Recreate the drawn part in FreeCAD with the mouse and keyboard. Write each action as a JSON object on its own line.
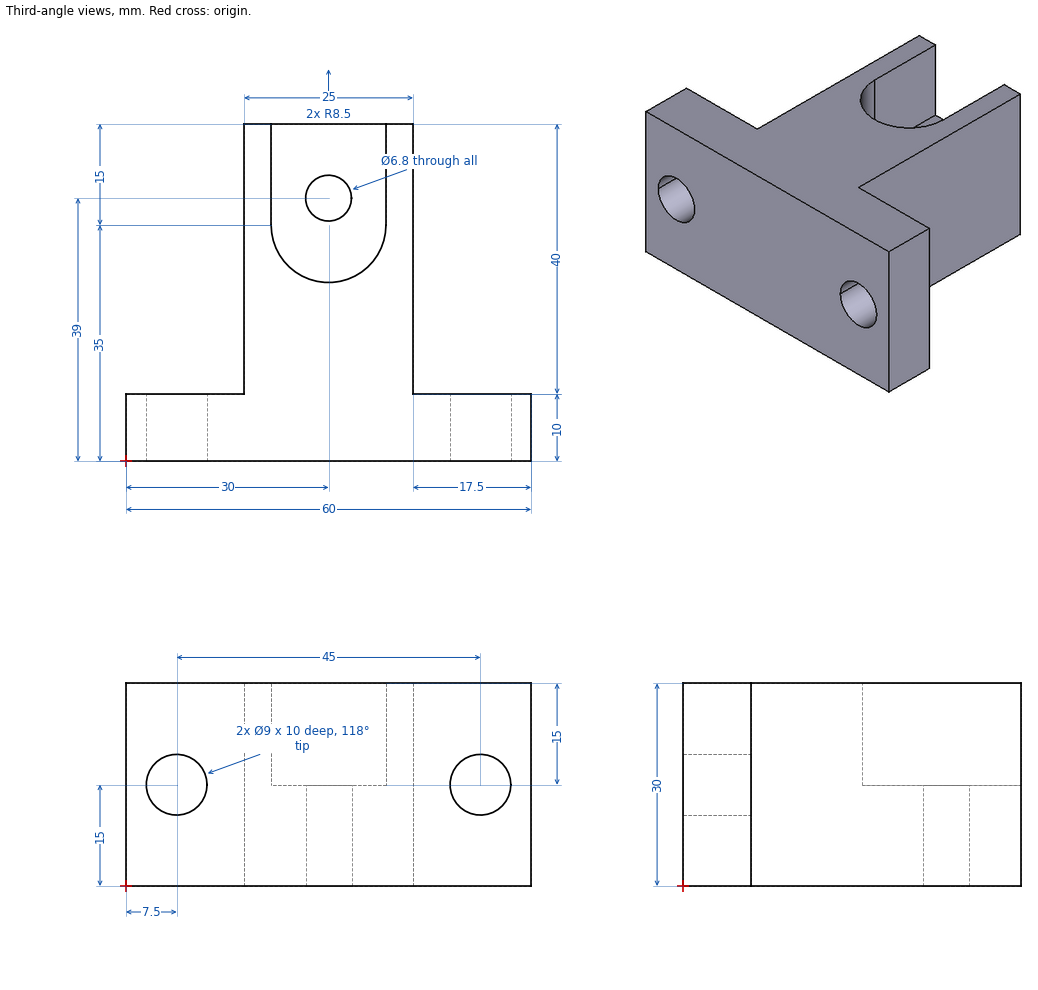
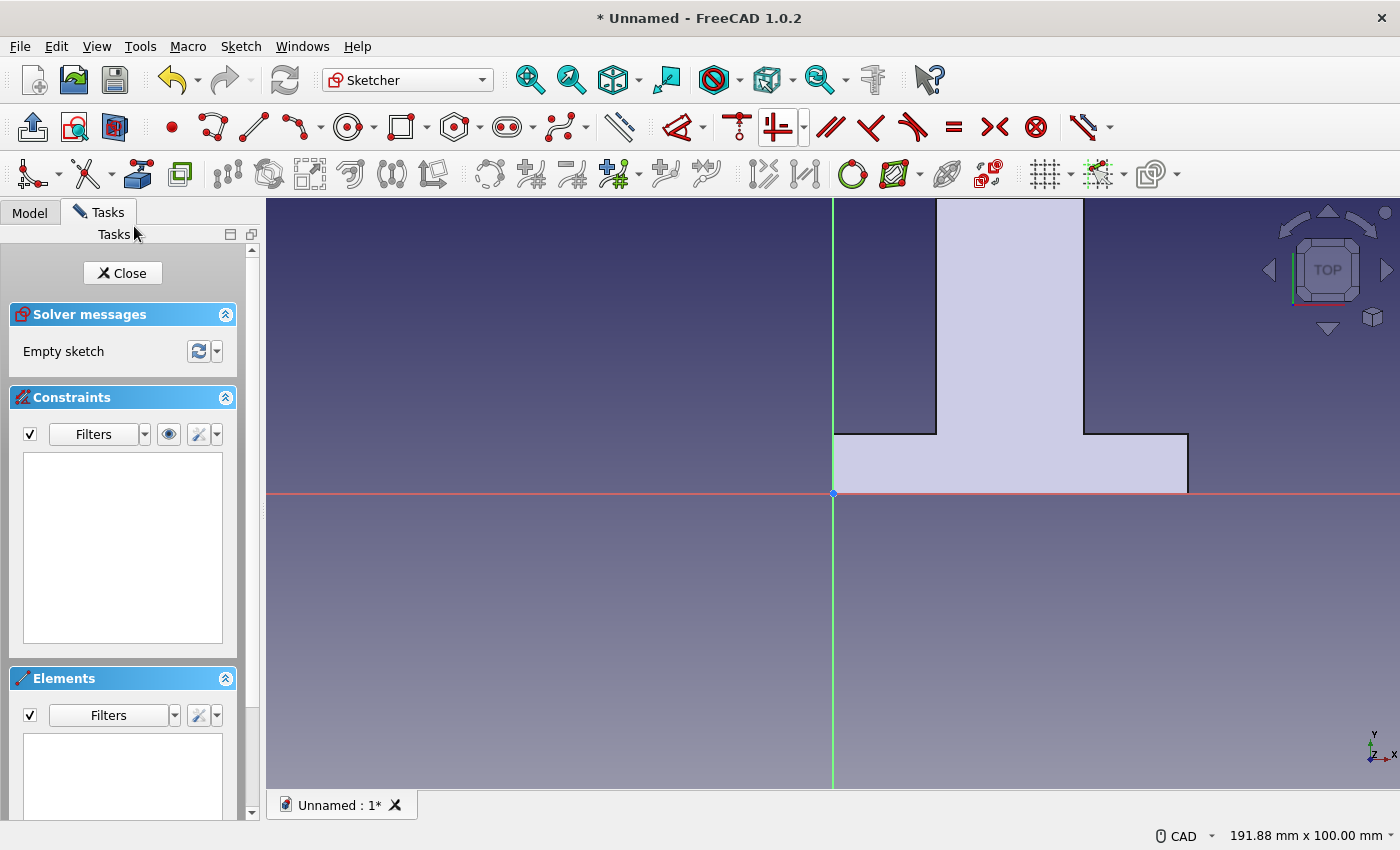
{"action": "scroll", "coordinate": [1041, 234], "scroll_direction": "up", "scroll_amount": 11}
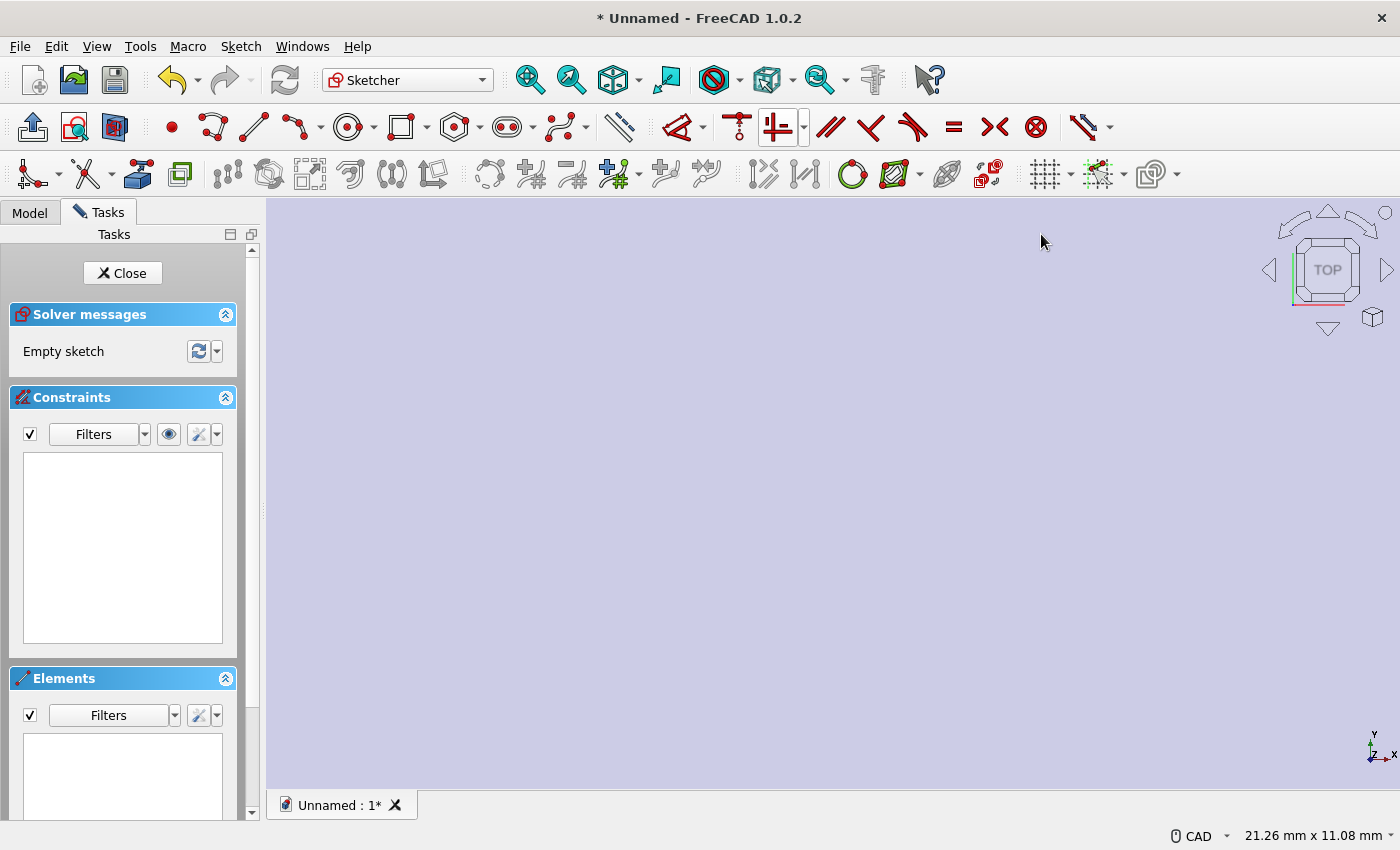
{"action": "key", "text": "g c"}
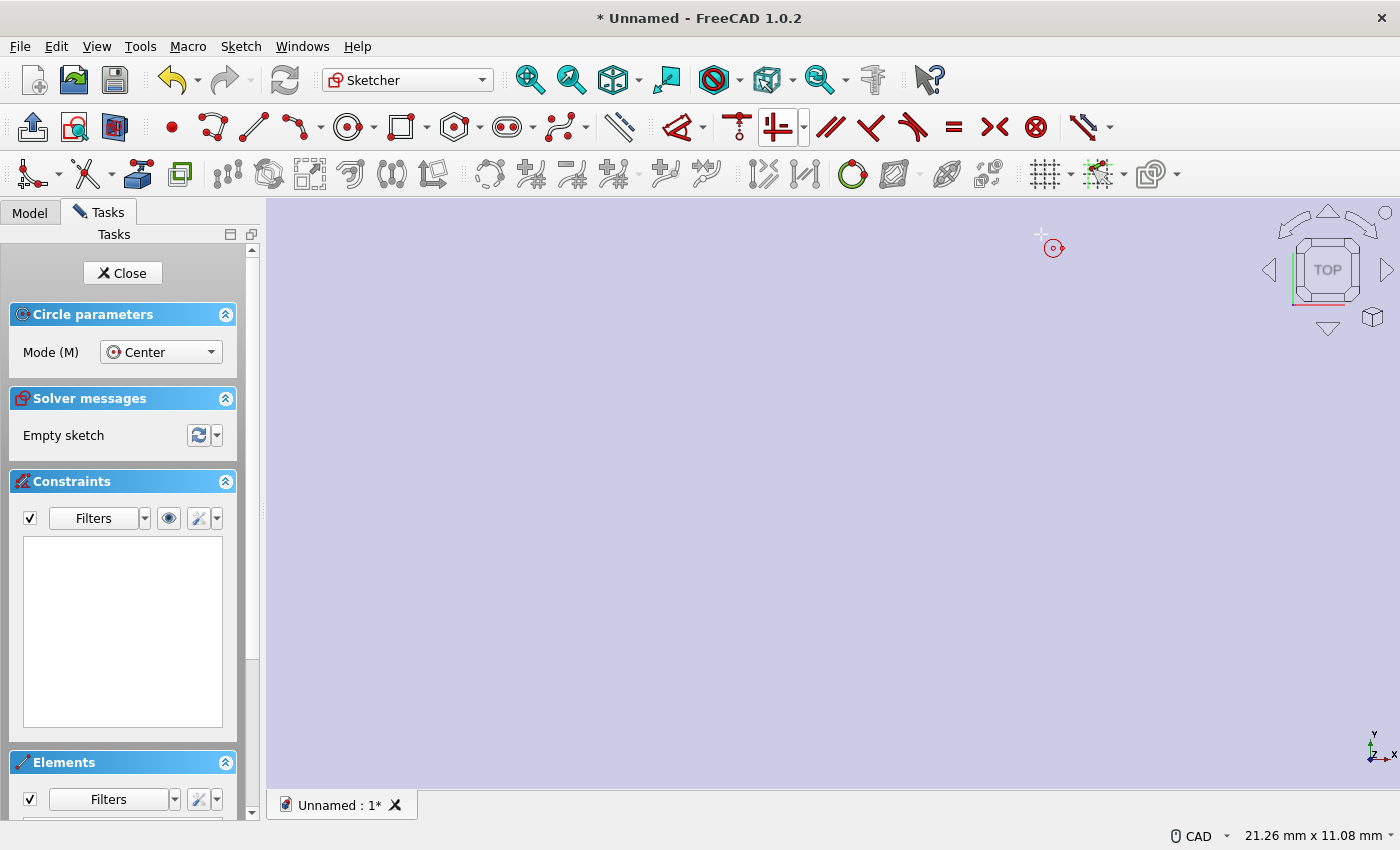
{"action": "left_click", "coordinate": [758, 495]}
{"action": "left_click", "coordinate": [887, 367]}
{"action": "key", "text": "Escape"}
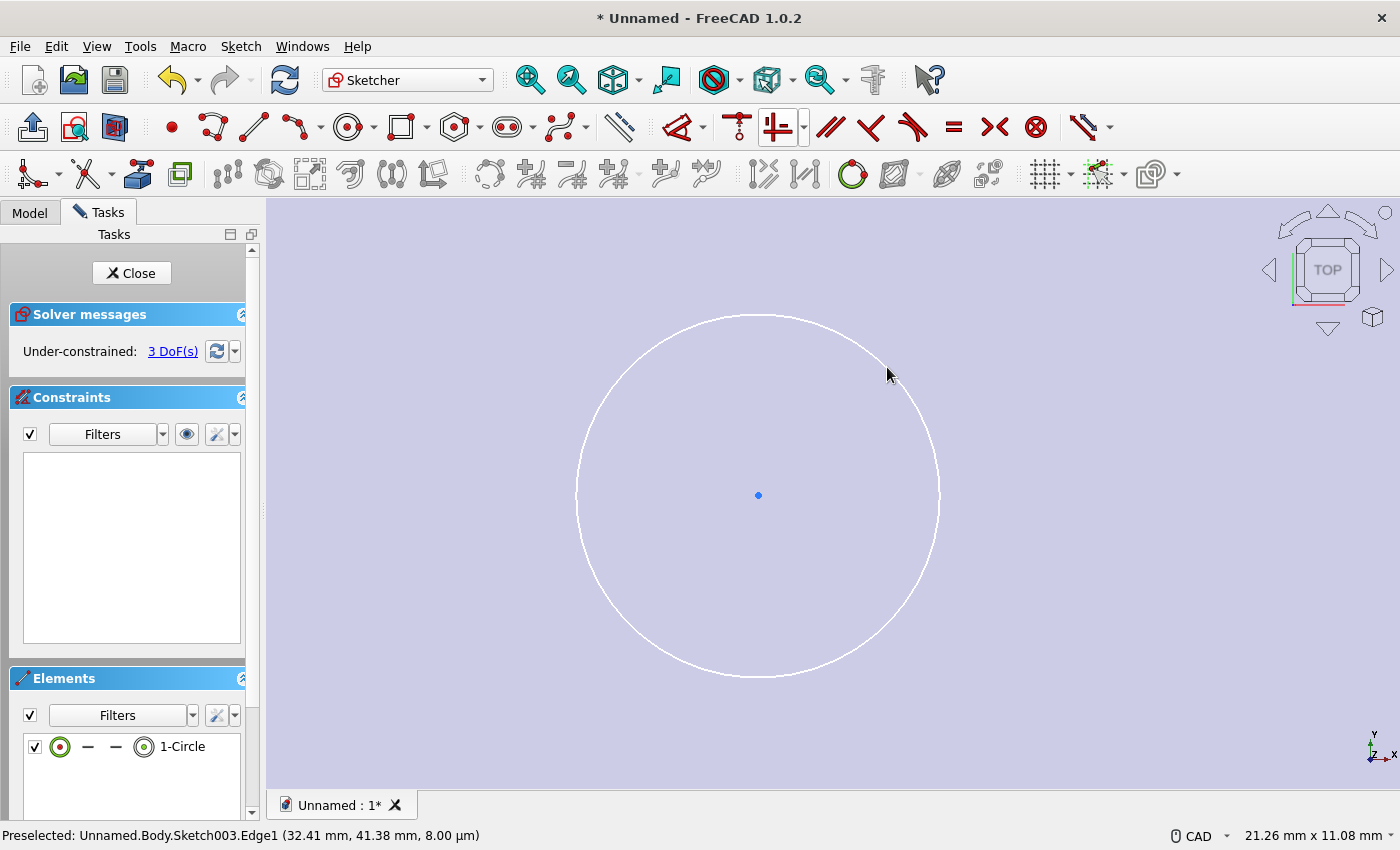
{"action": "left_click", "coordinate": [676, 128]}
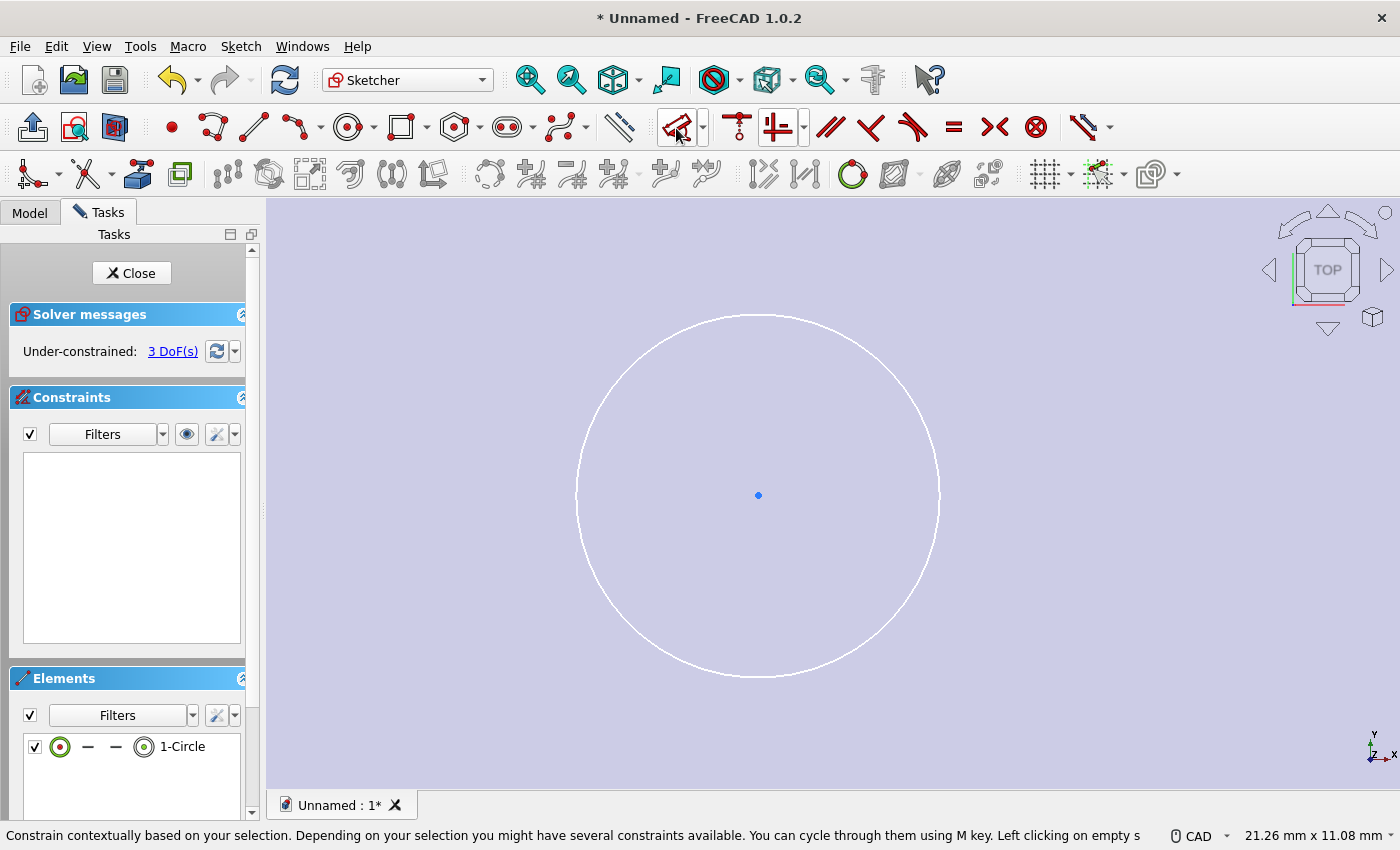
{"action": "left_click", "coordinate": [886, 367]}
{"action": "left_click", "coordinate": [909, 344]}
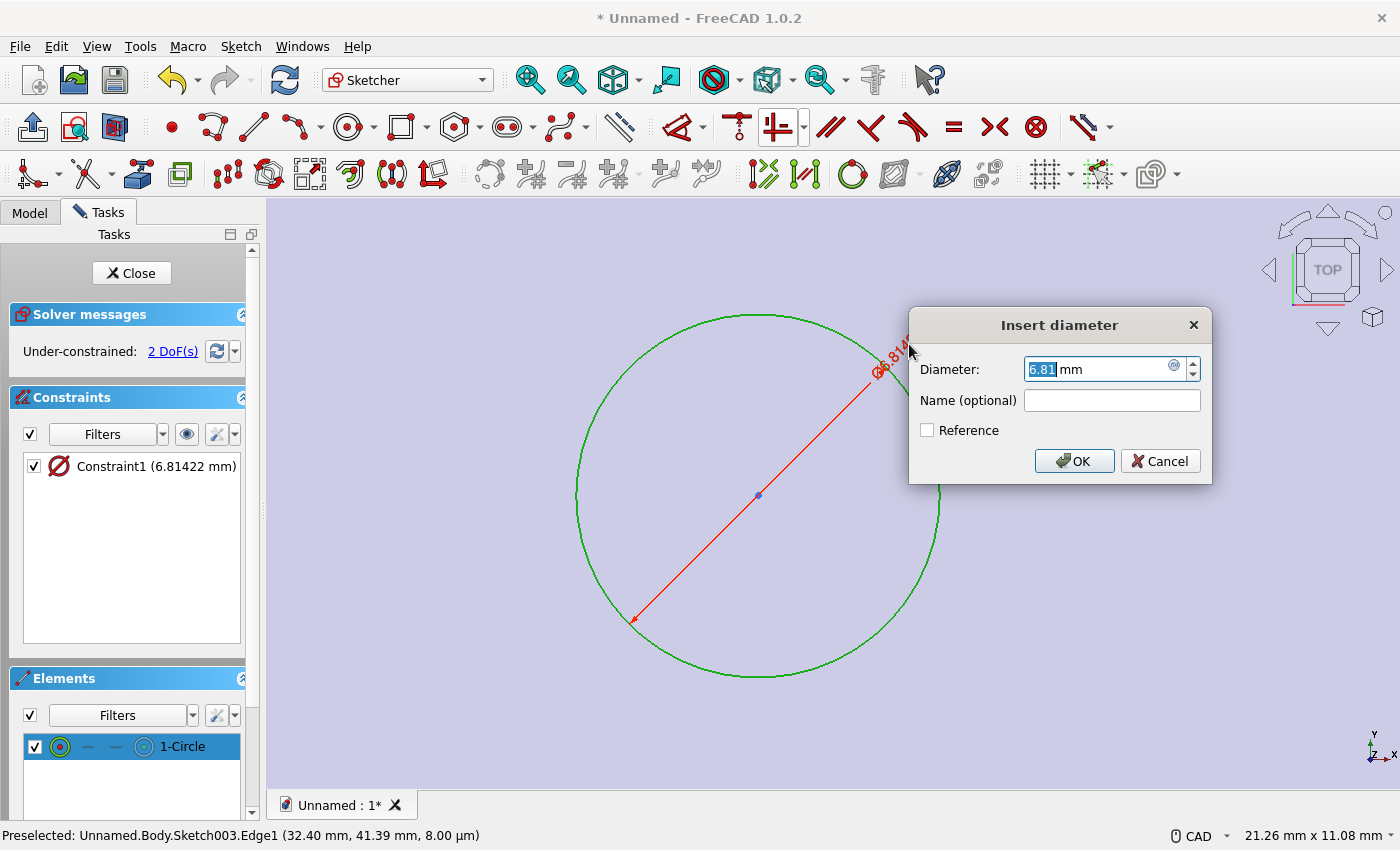
{"action": "type", "text": "6.8"}
{"action": "key", "text": "Return"}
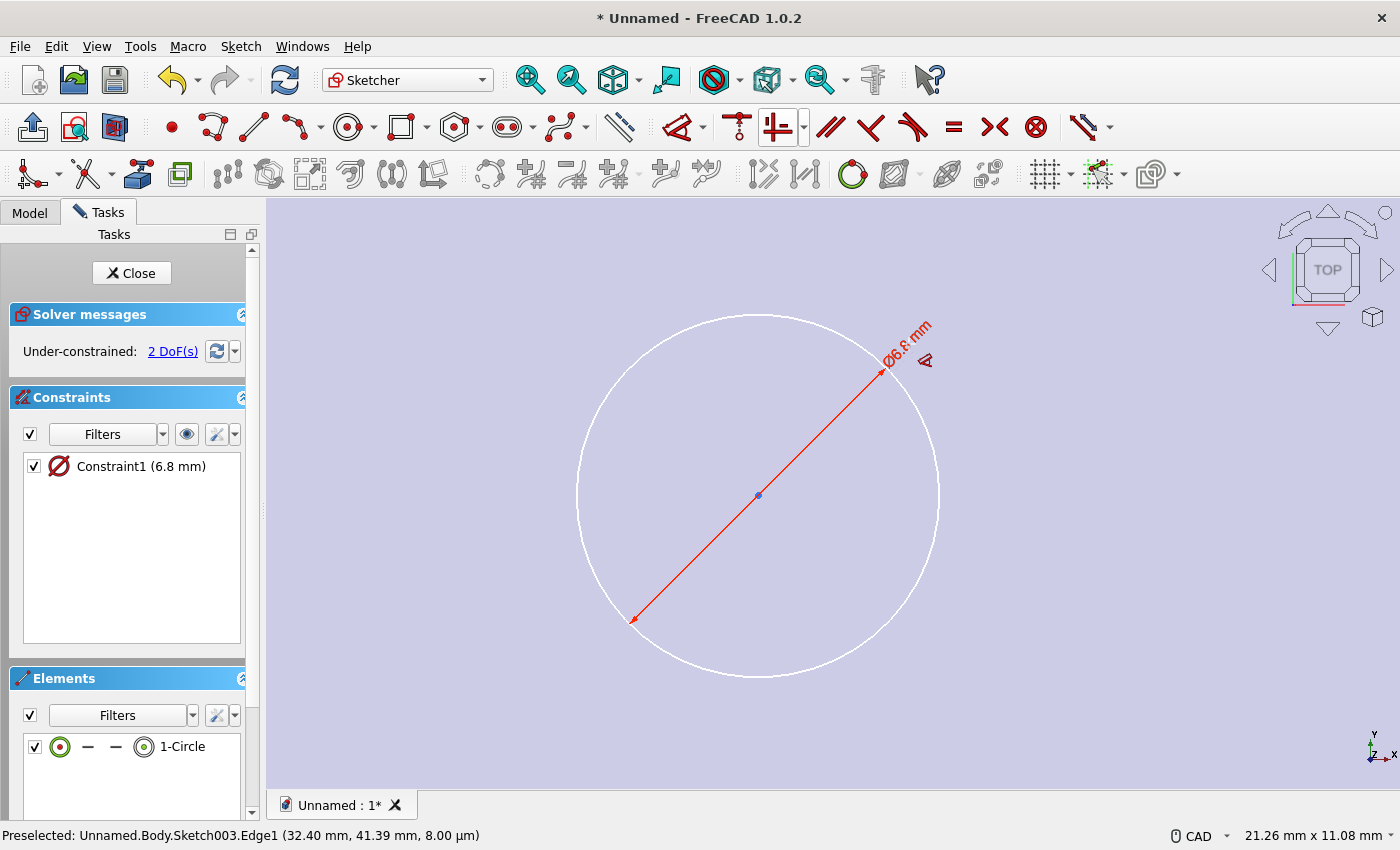
{"action": "left_click", "coordinate": [758, 496]}
{"action": "left_click", "coordinate": [526, 462]}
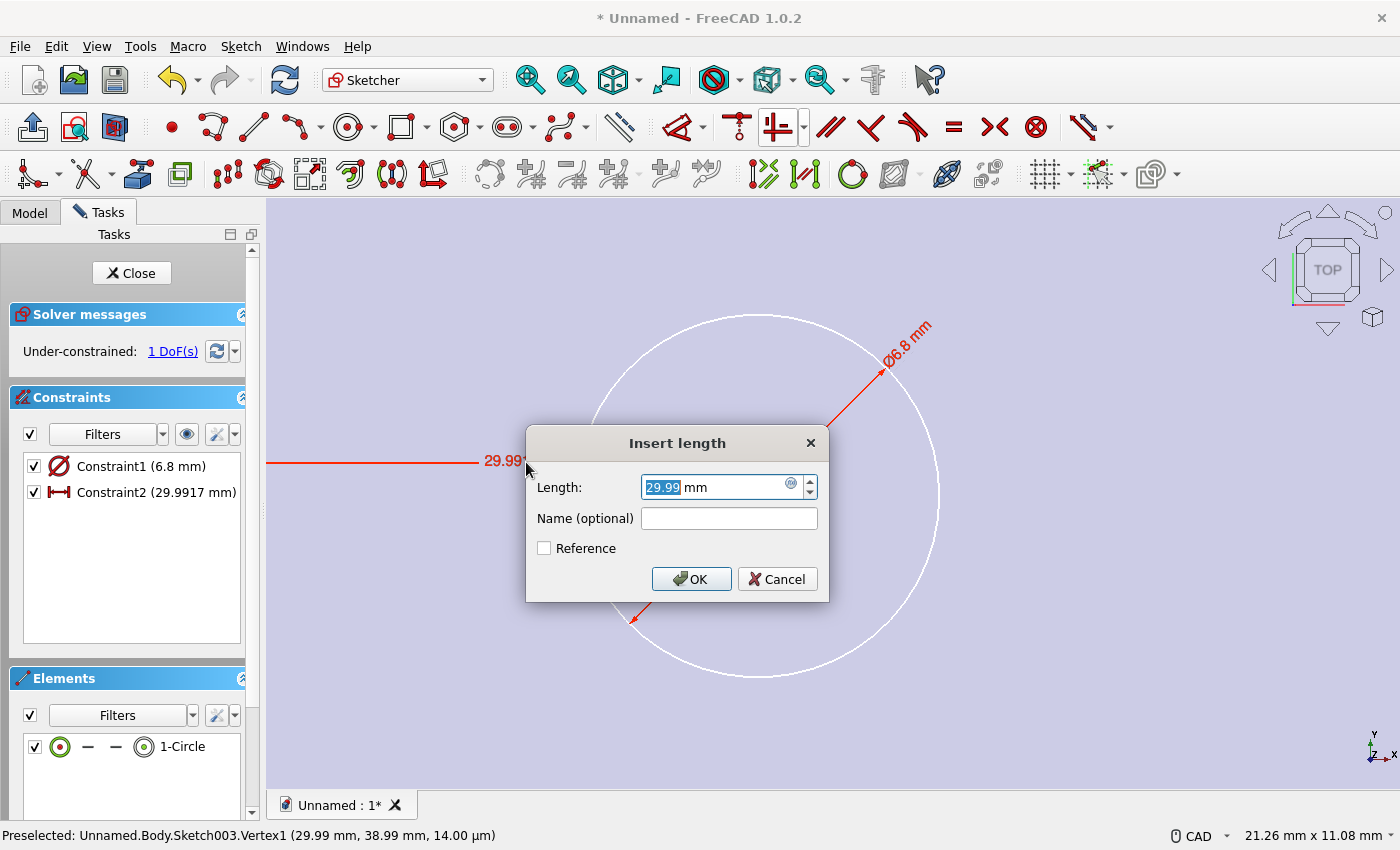
{"action": "type", "text": "30"}
{"action": "key", "text": "Return"}